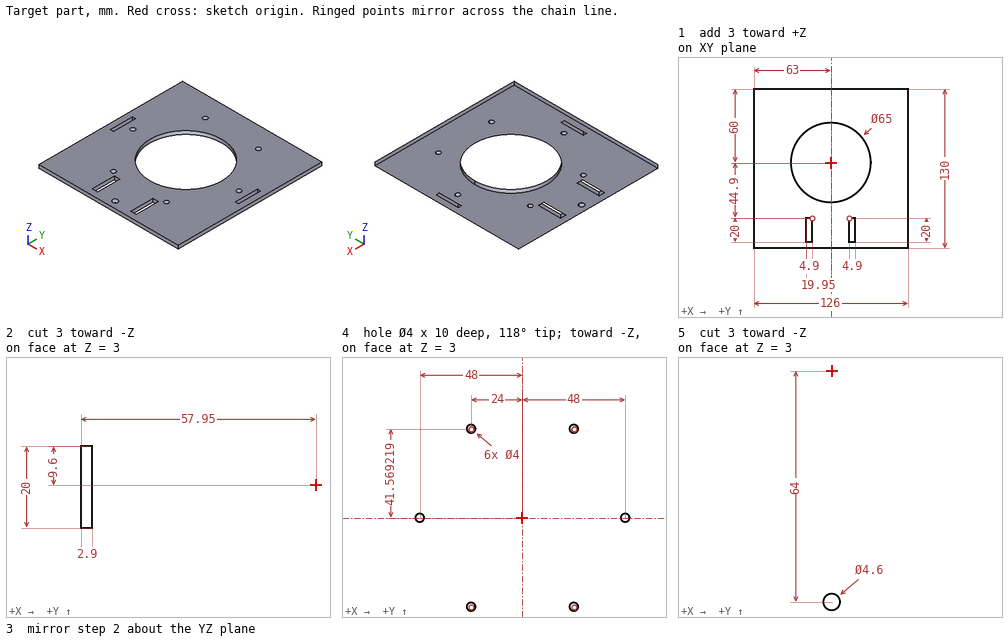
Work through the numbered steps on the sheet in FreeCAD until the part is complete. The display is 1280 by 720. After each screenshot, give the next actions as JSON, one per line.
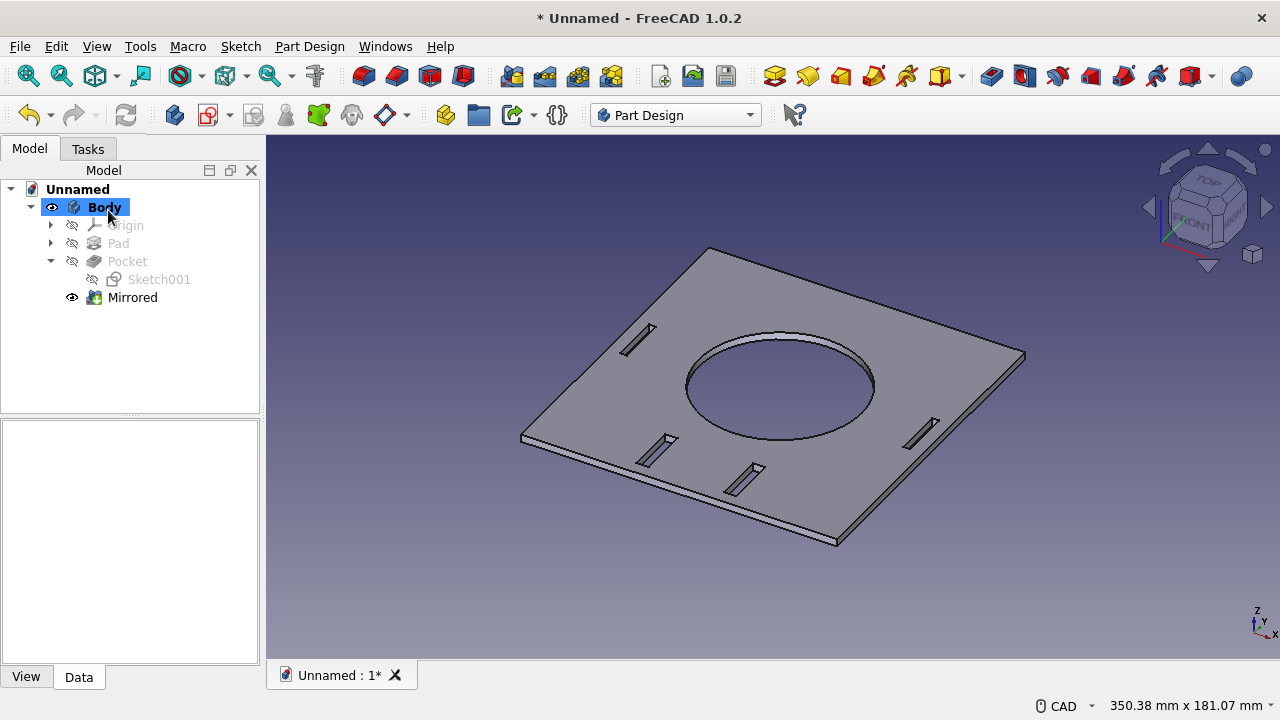
{"action": "left_click", "coordinate": [809, 476]}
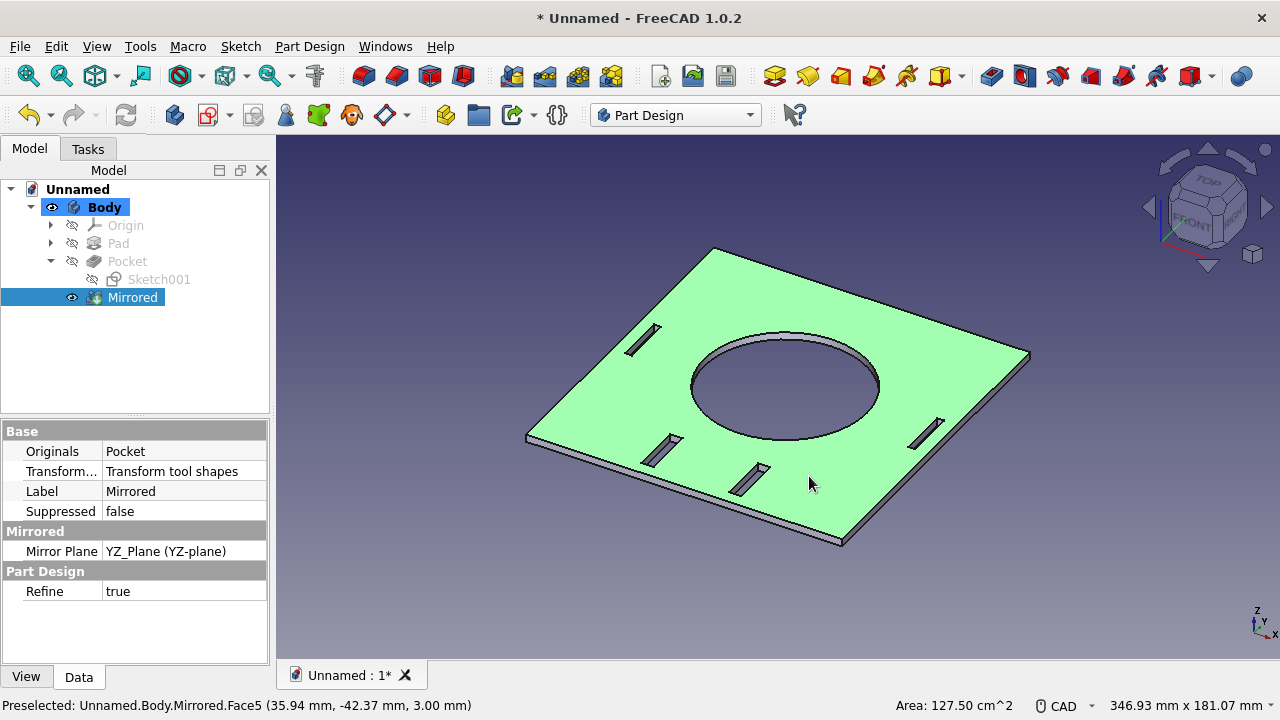
{"action": "left_click", "coordinate": [208, 116]}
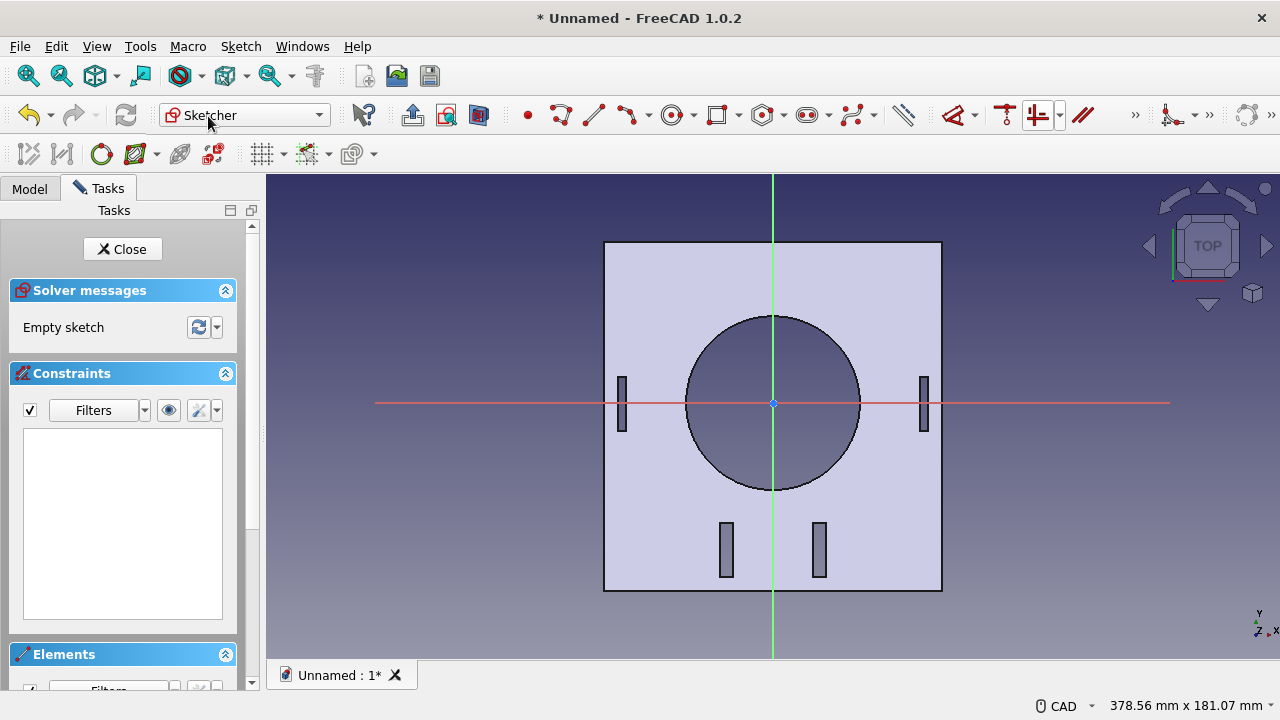
{"action": "left_click", "coordinate": [672, 116]}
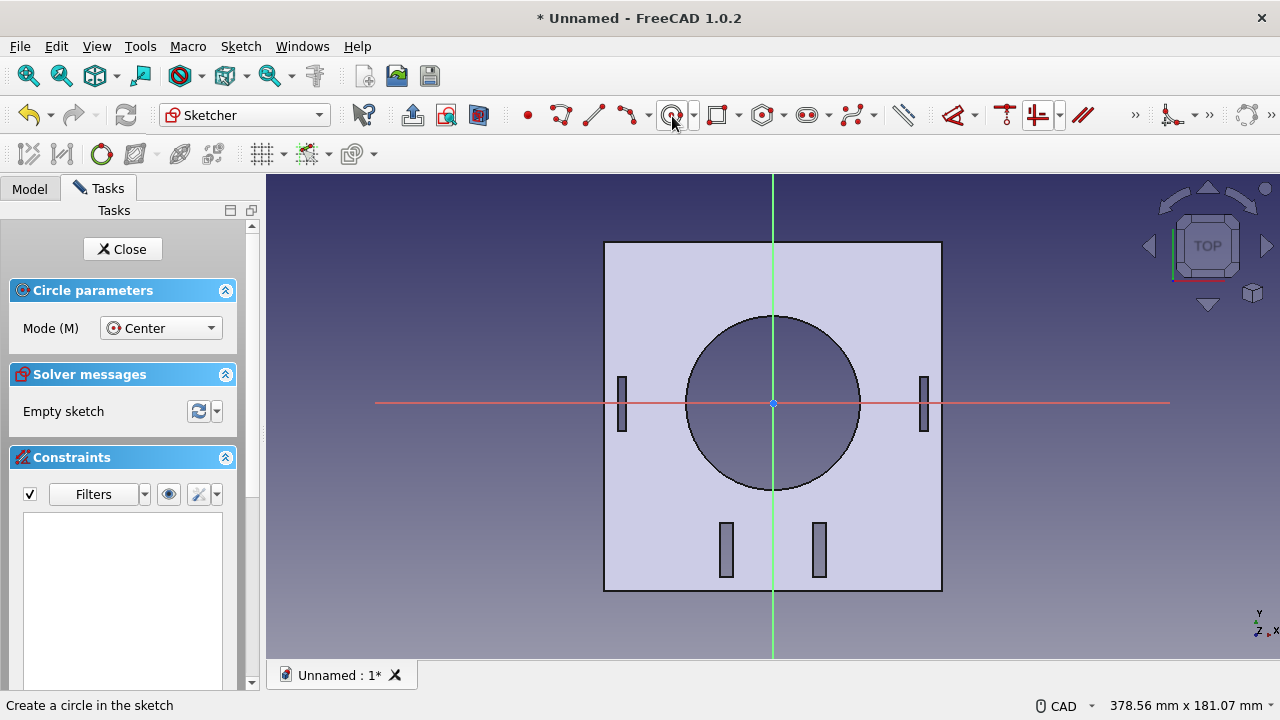
{"action": "scroll", "coordinate": [709, 292], "scroll_direction": "up", "scroll_amount": 8}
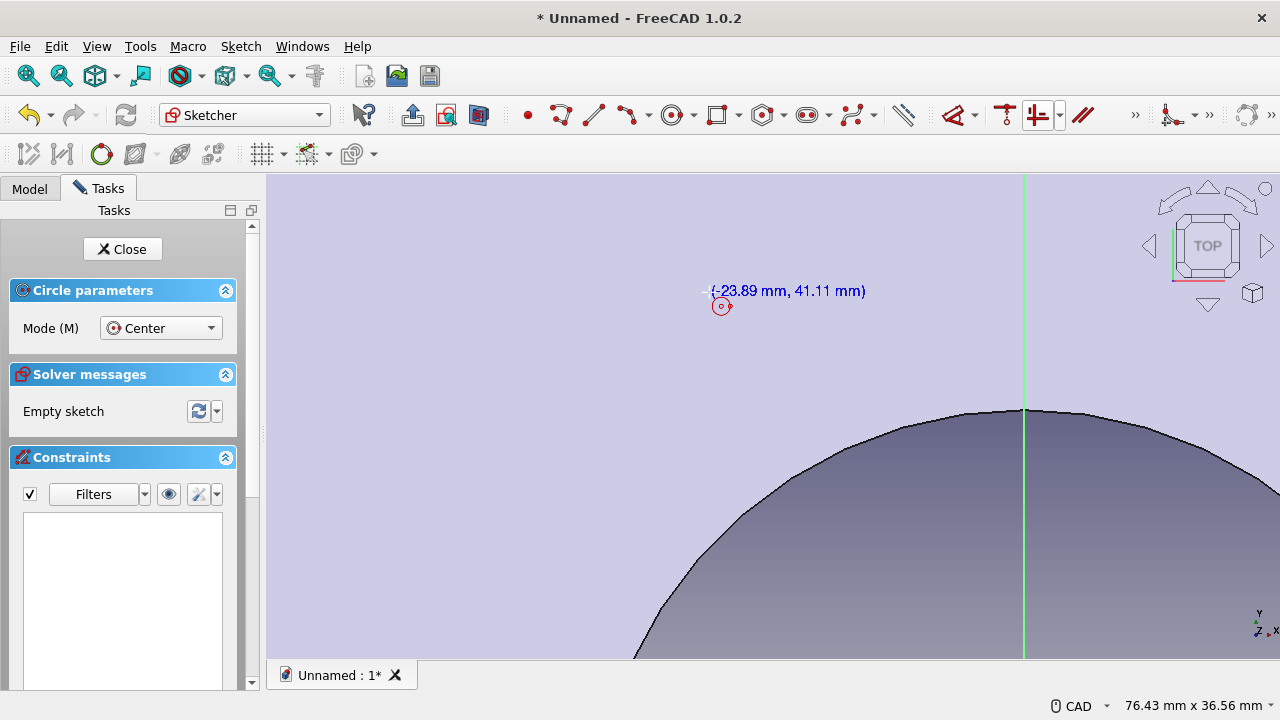
{"action": "scroll", "coordinate": [600, 277], "scroll_direction": "down", "scroll_amount": 7}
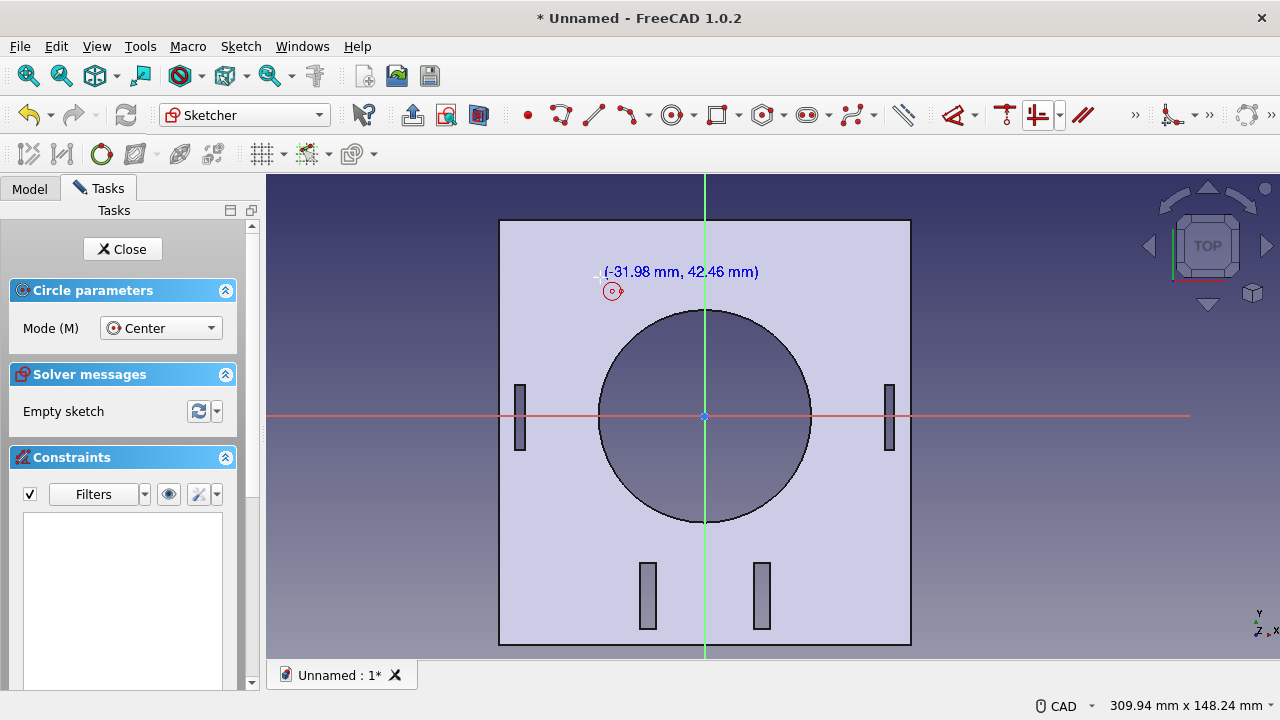
{"action": "left_click", "coordinate": [626, 280]}
{"action": "mouse_move", "coordinate": [631, 276]}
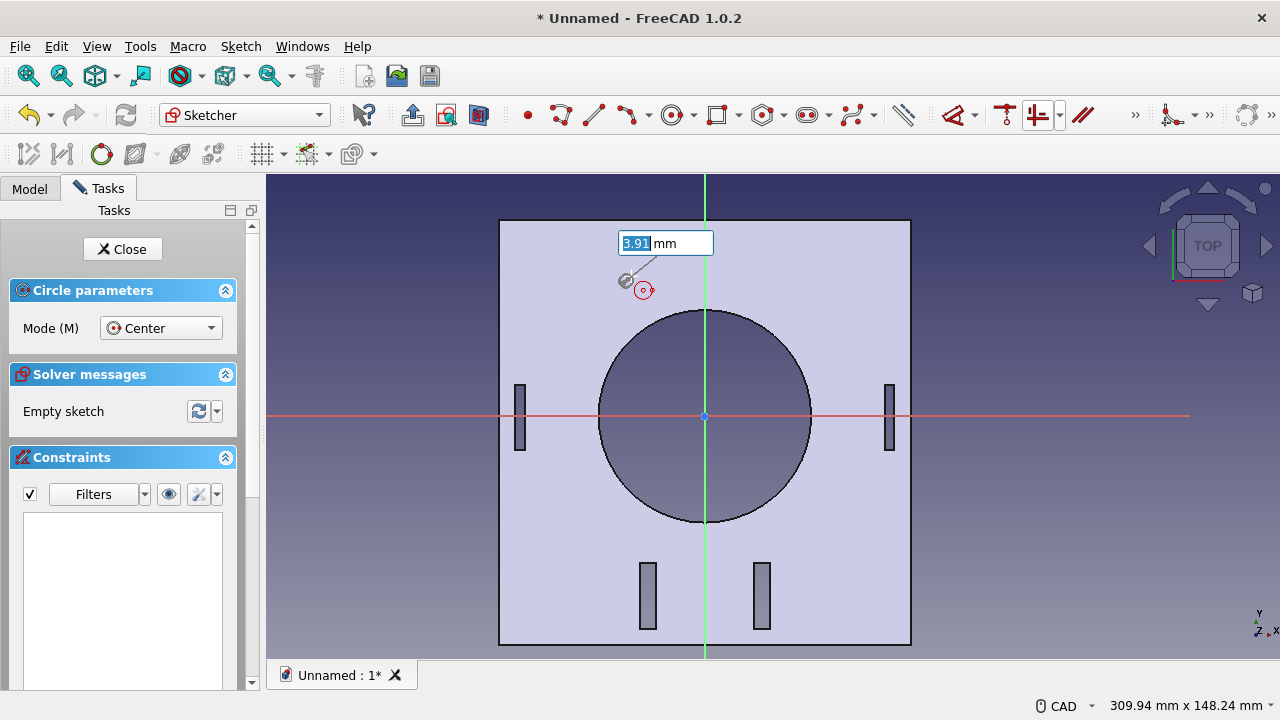
{"action": "type", "text": "4"}
{"action": "key", "text": "Return"}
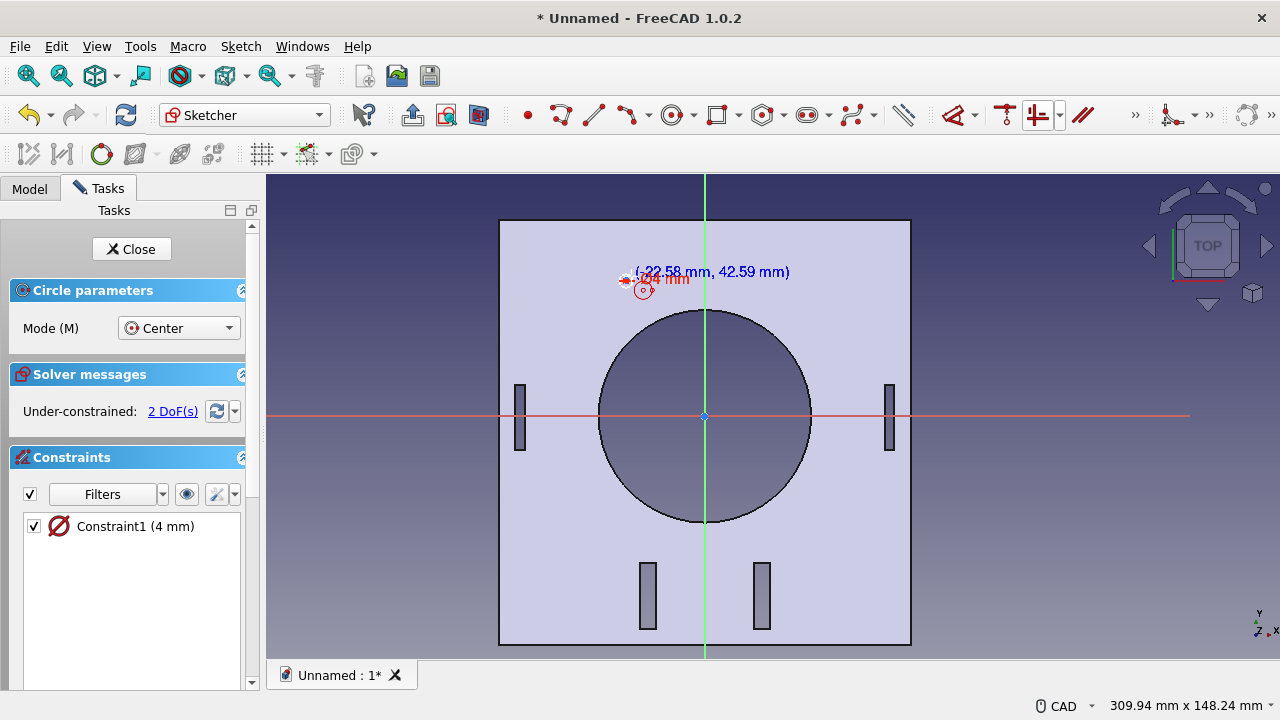
{"action": "scroll", "coordinate": [862, 416], "scroll_direction": "up", "scroll_amount": 7}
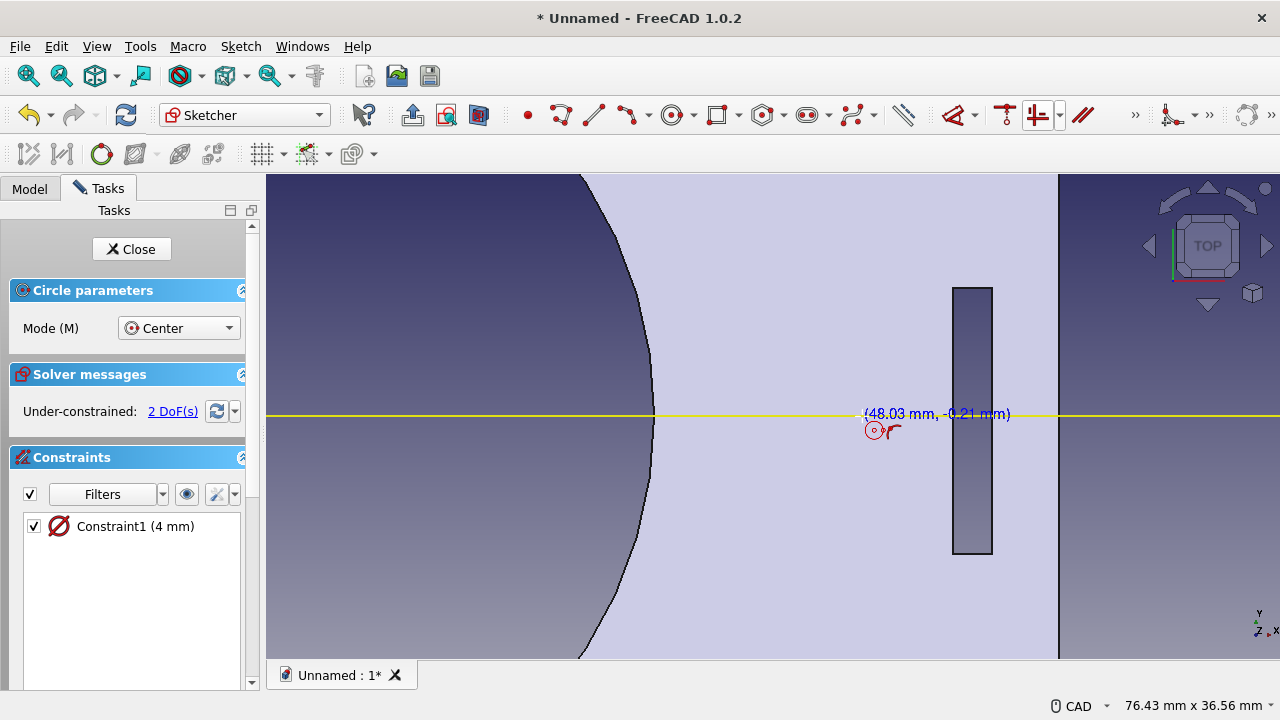
{"action": "scroll", "coordinate": [862, 417], "scroll_direction": "down", "scroll_amount": 7}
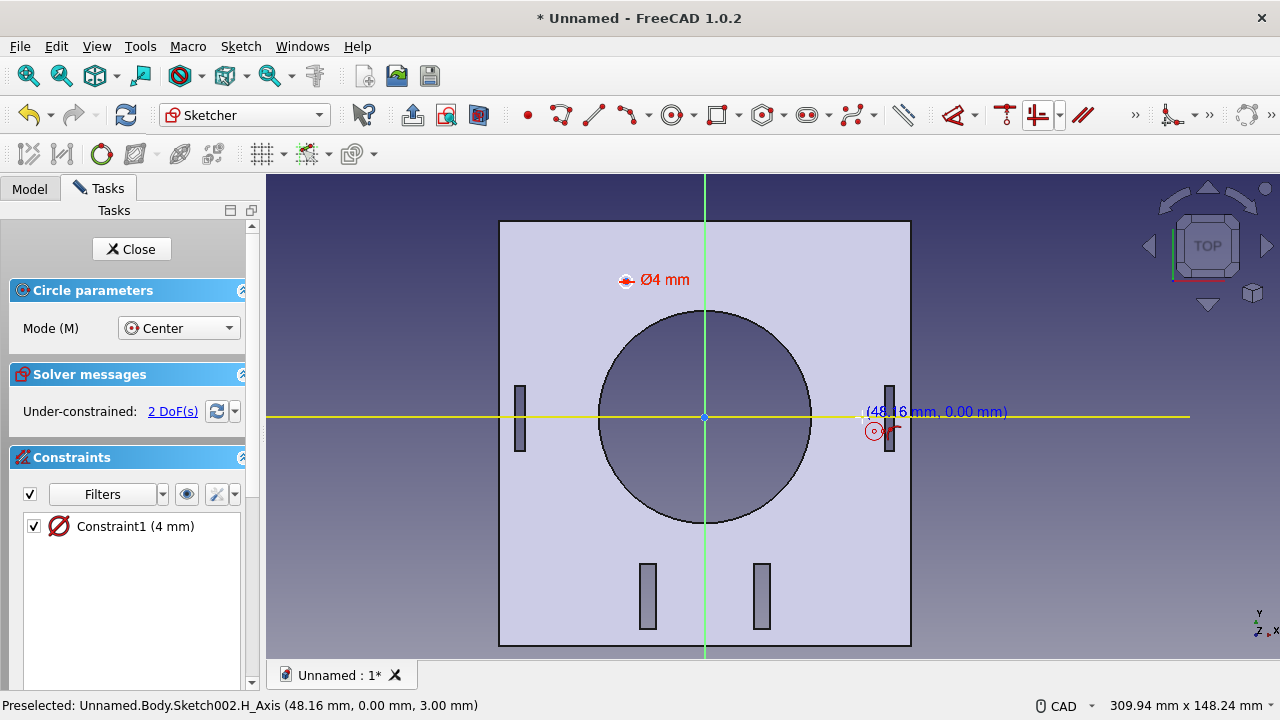
{"action": "left_click", "coordinate": [862, 417]}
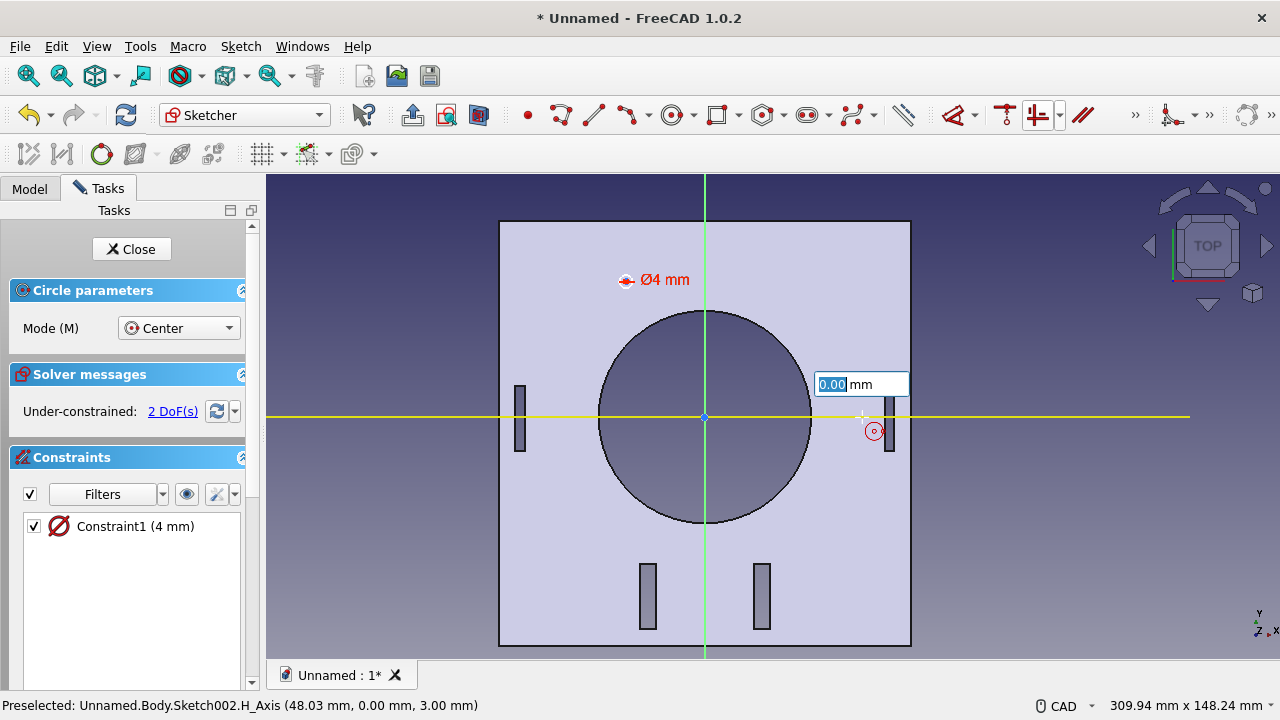
{"action": "scroll", "coordinate": [860, 423], "scroll_direction": "up", "scroll_amount": 5}
{"action": "mouse_move", "coordinate": [858, 423]}